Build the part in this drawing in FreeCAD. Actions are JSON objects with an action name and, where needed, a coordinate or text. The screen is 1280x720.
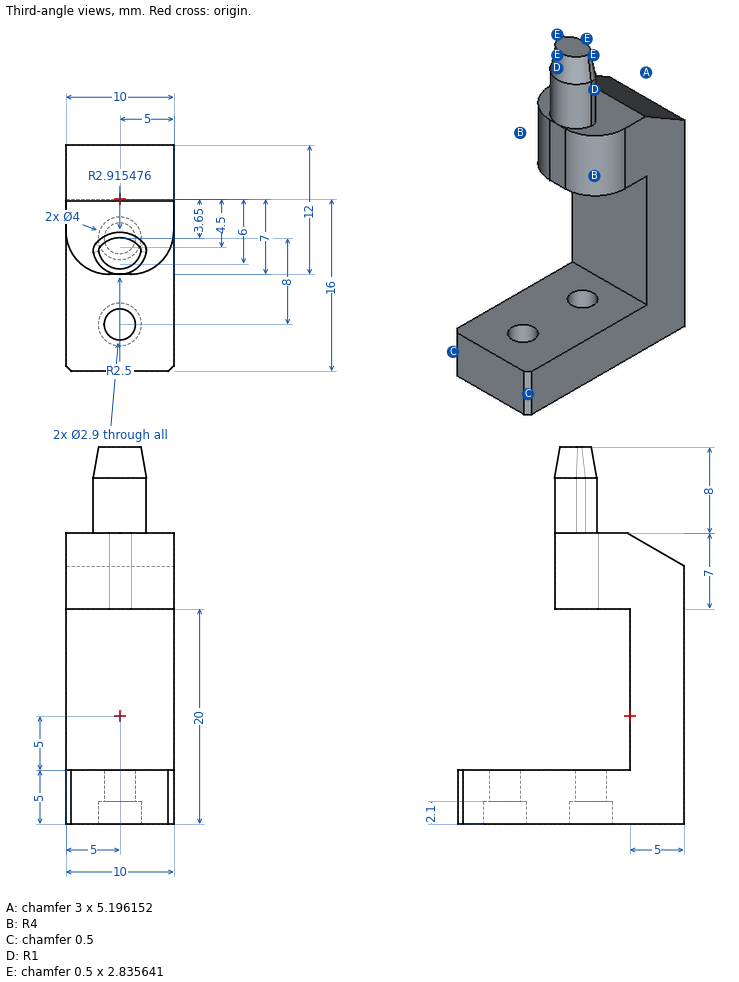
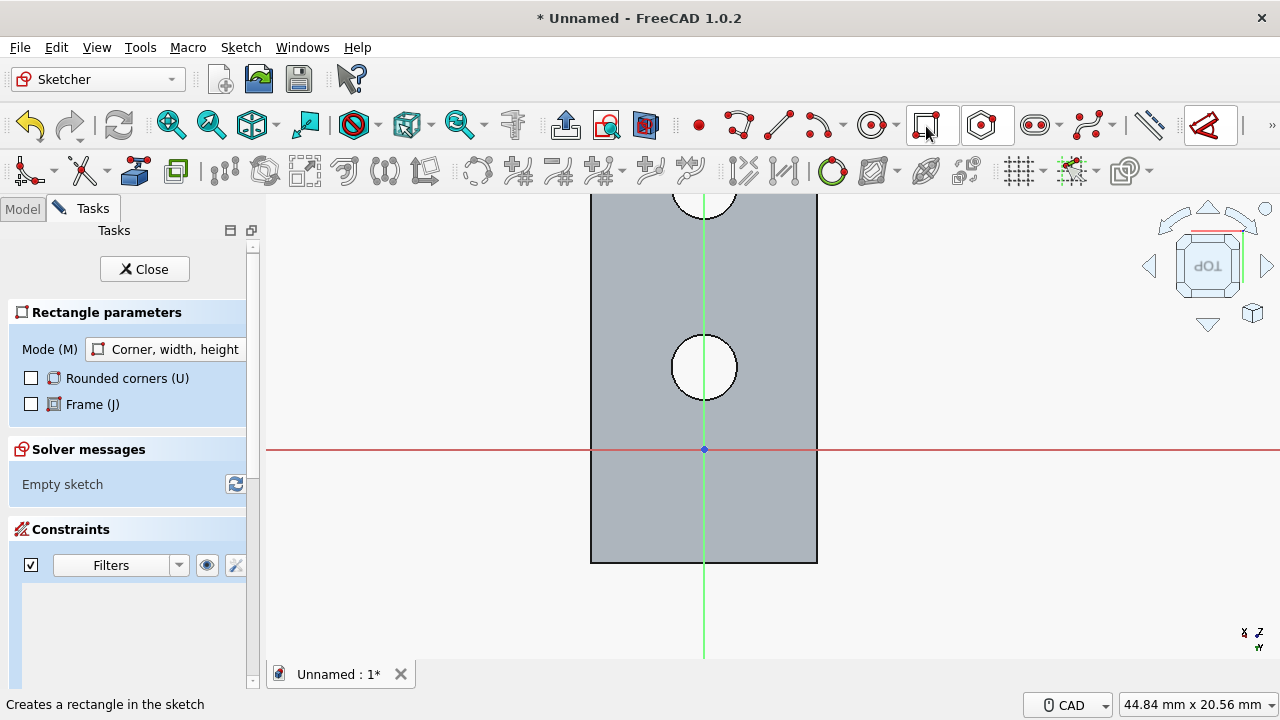
{"action": "left_click", "coordinate": [591, 292]}
{"action": "left_click", "coordinate": [817, 563]}
{"action": "key", "text": "Escape"}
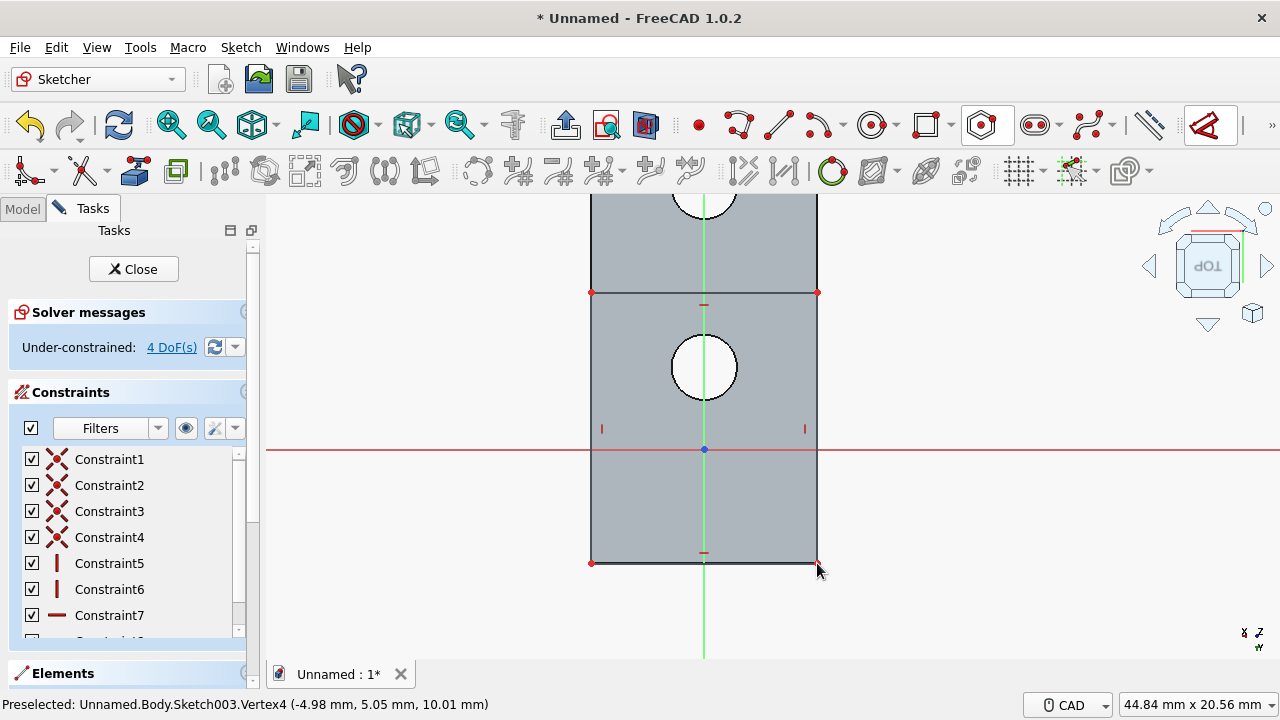
{"action": "left_click", "coordinate": [1204, 126]}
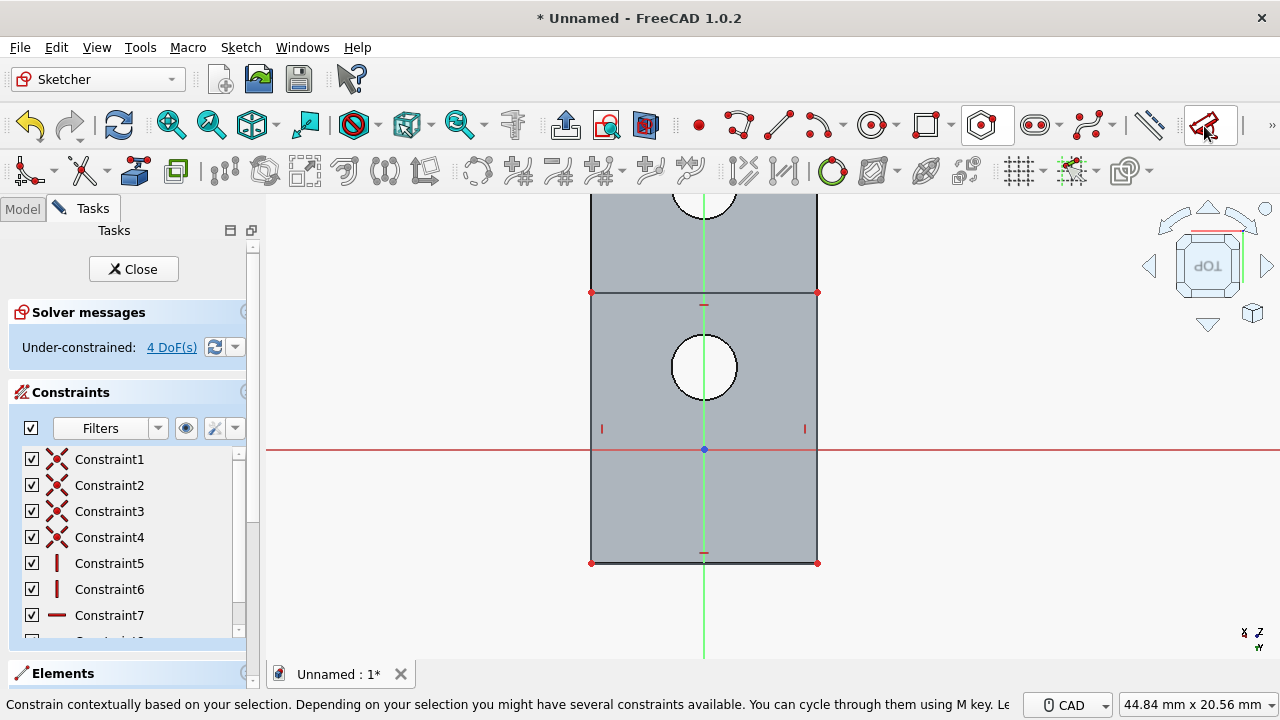
{"action": "left_click", "coordinate": [591, 374]}
{"action": "left_click", "coordinate": [557, 428]}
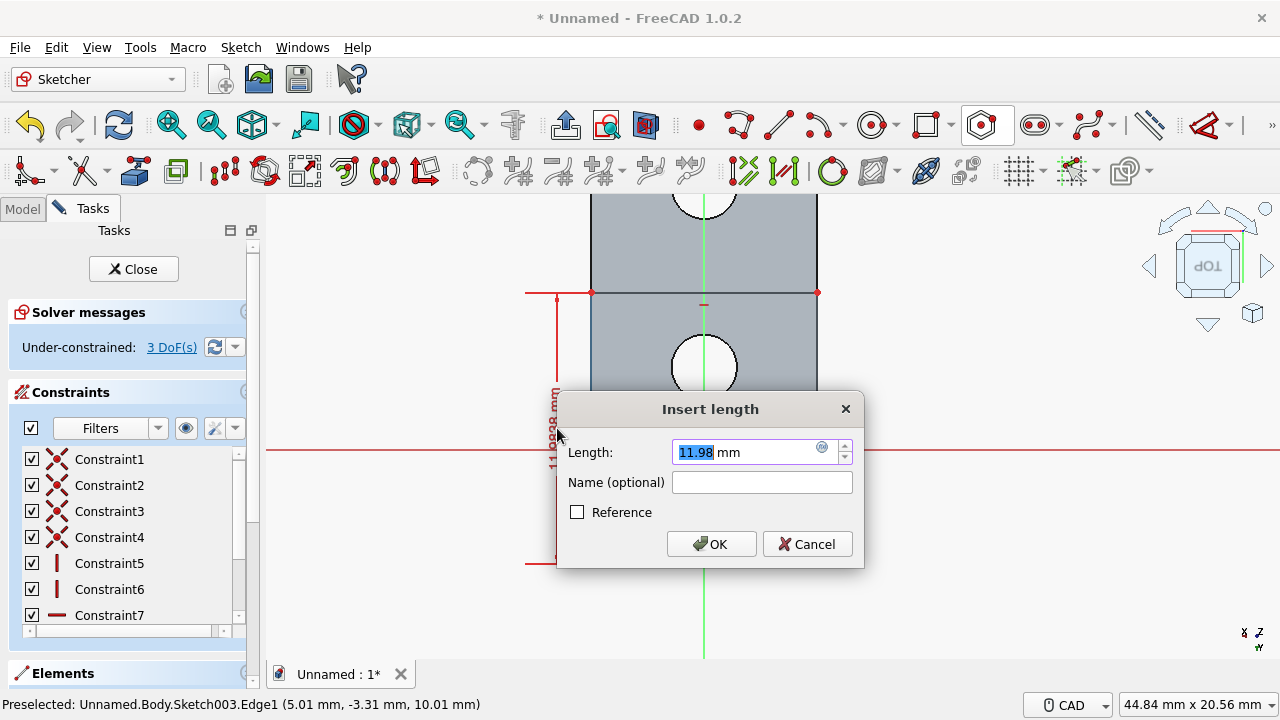
{"action": "type", "text": "12"}
{"action": "key", "text": "Return"}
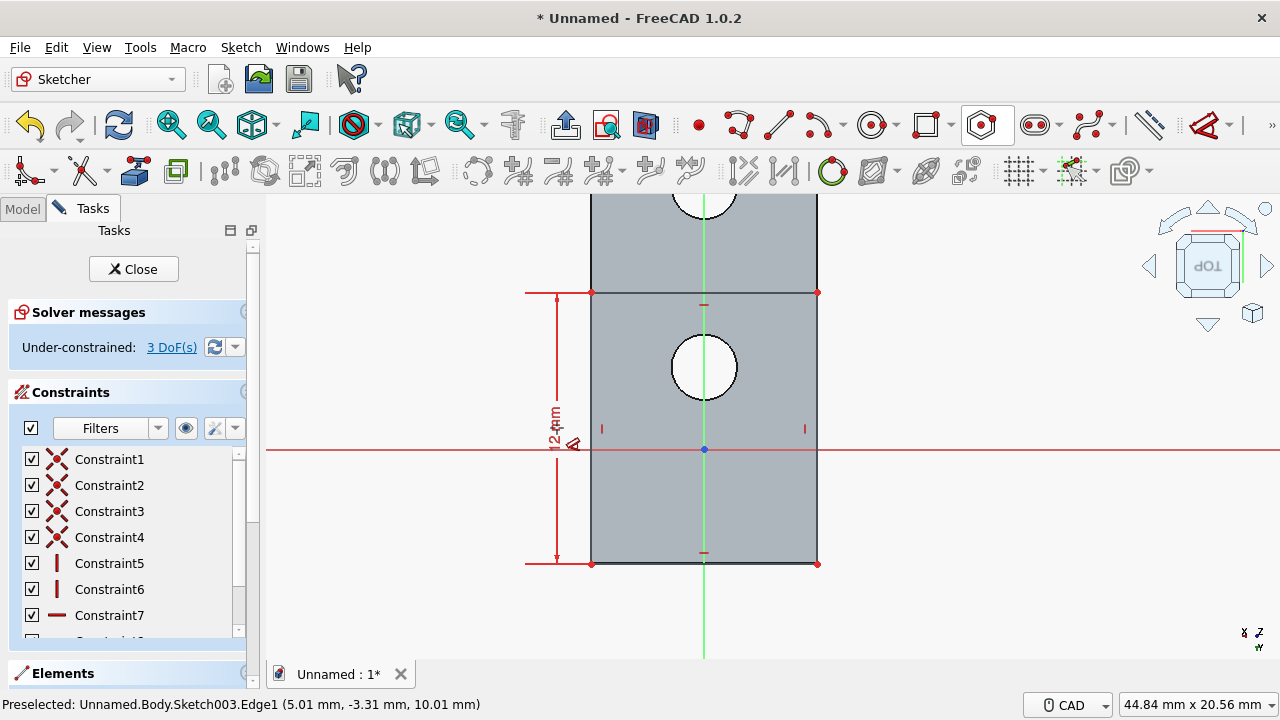
{"action": "left_click", "coordinate": [659, 564]}
{"action": "left_click", "coordinate": [652, 598]}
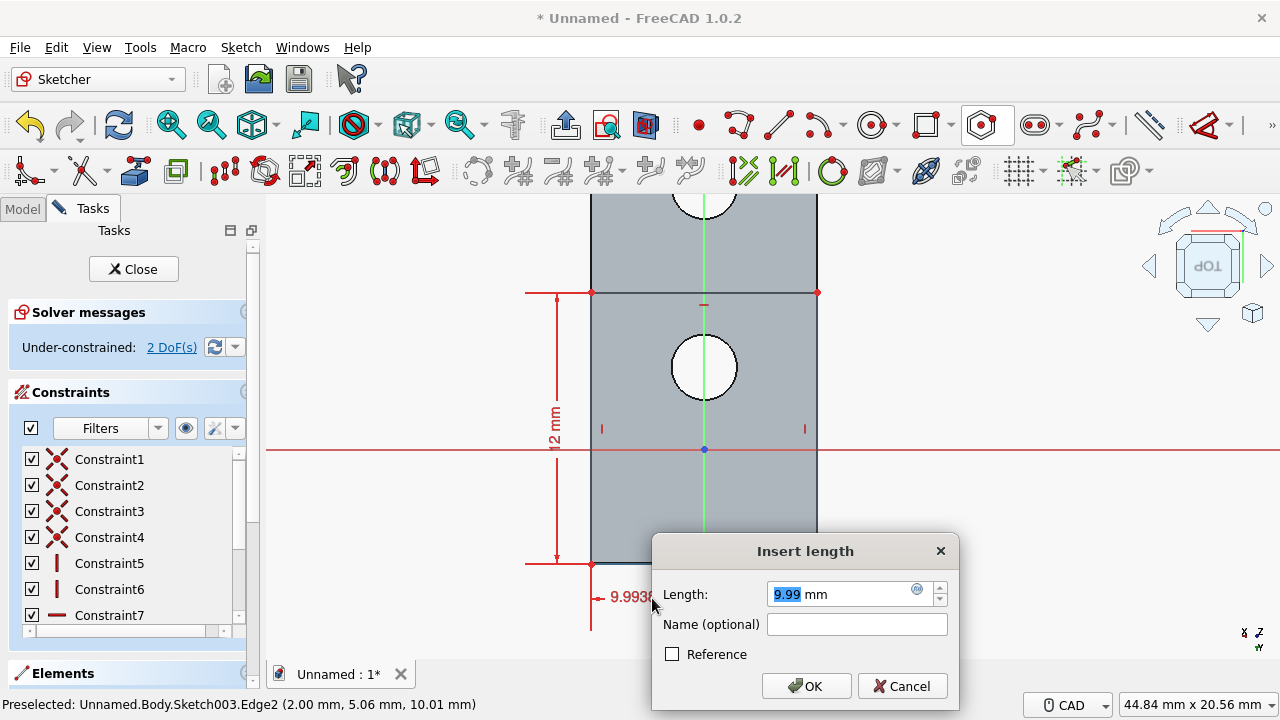
{"action": "type", "text": "10"}
{"action": "key", "text": "Return"}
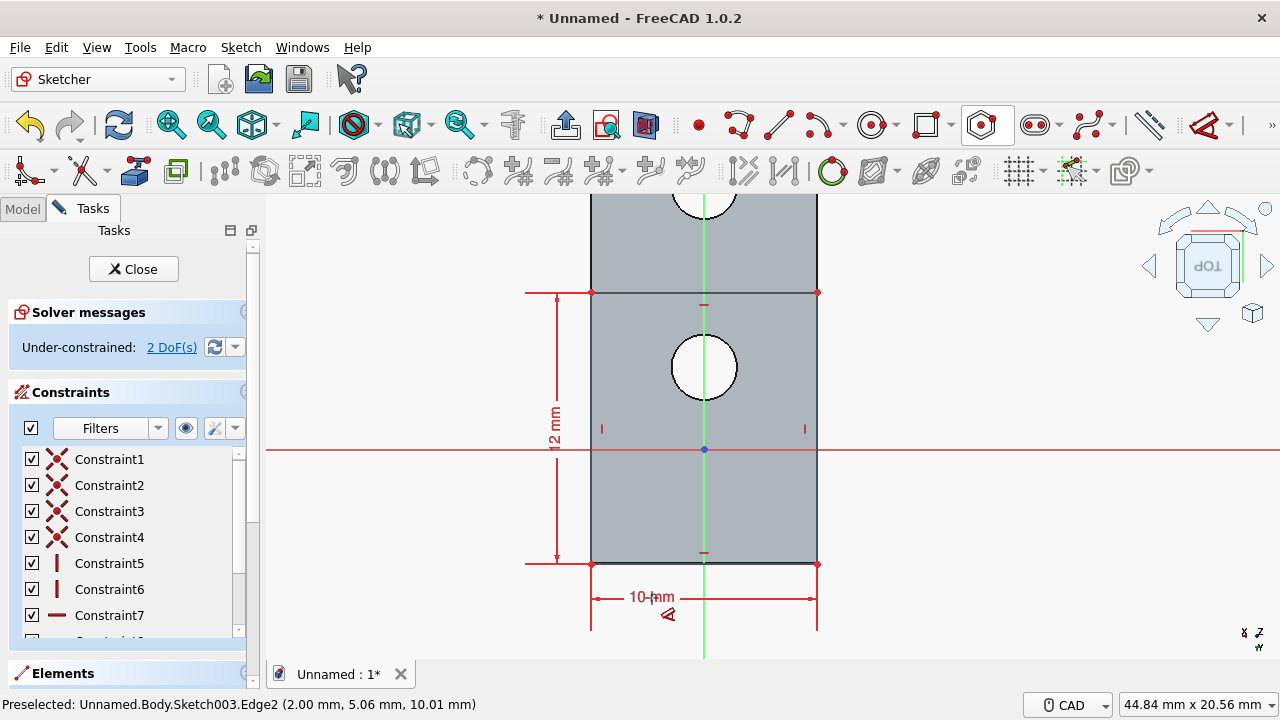
{"action": "left_click", "coordinate": [591, 293]}
{"action": "left_click", "coordinate": [648, 259]}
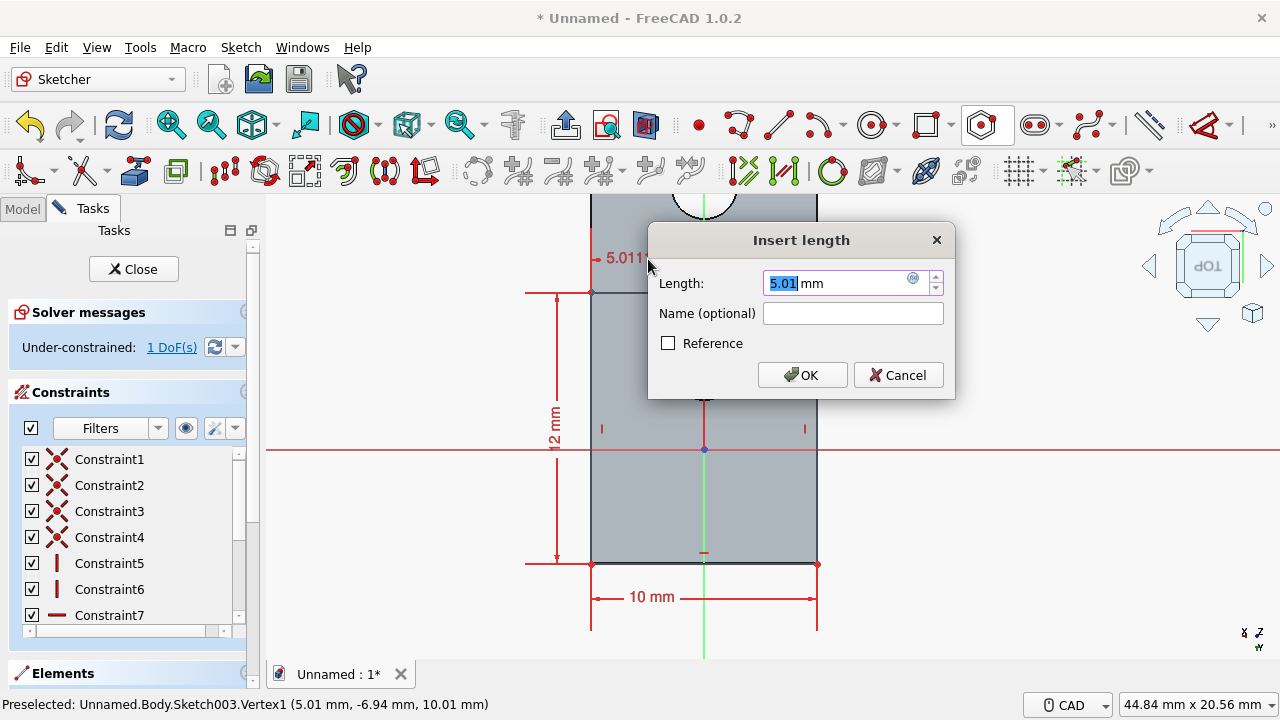
{"action": "type", "text": "5"}
{"action": "key", "text": "Return"}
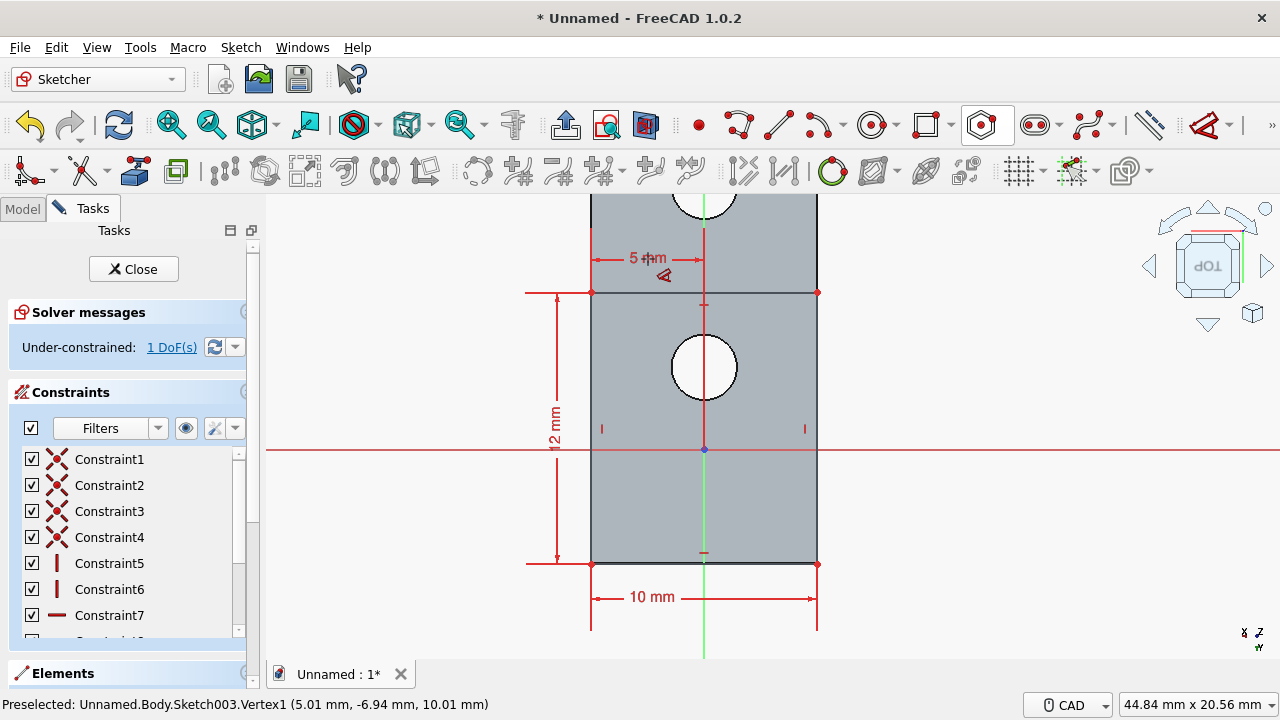
{"action": "left_click", "coordinate": [591, 293]}
{"action": "left_click", "coordinate": [557, 371]}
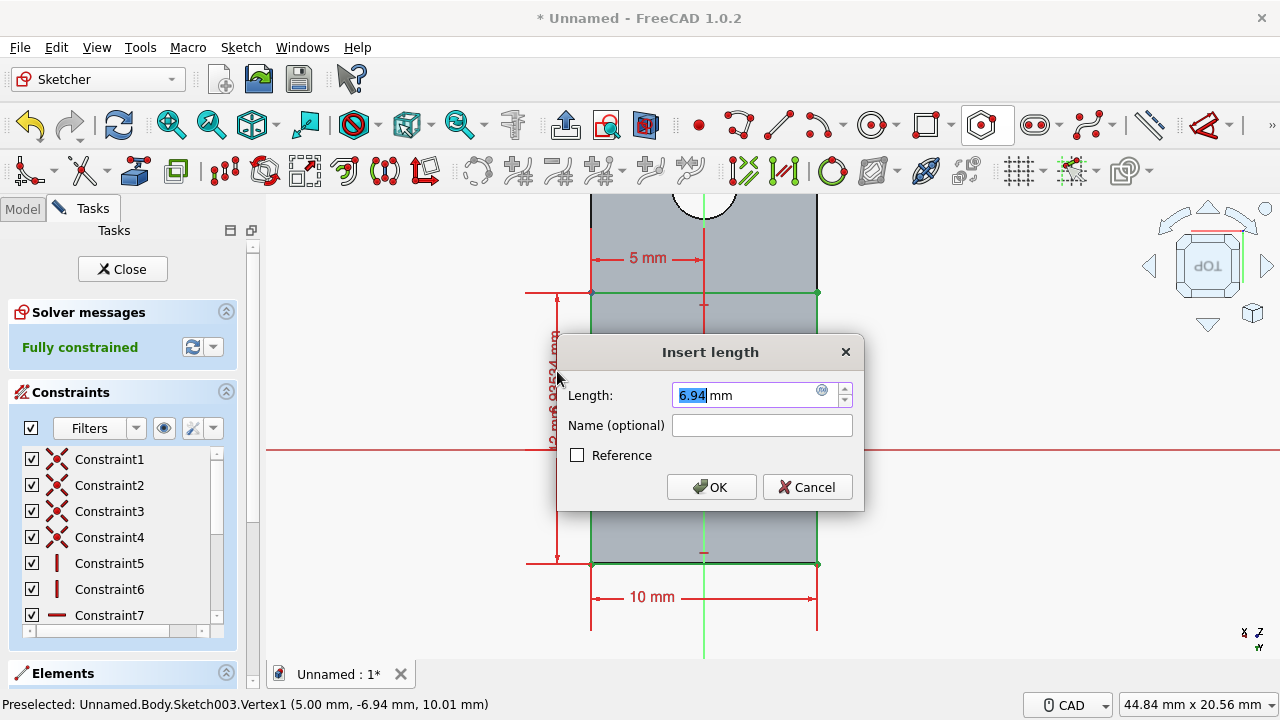
{"action": "type", "text": "7"}
{"action": "key", "text": "Return"}
{"action": "key", "text": "Escape"}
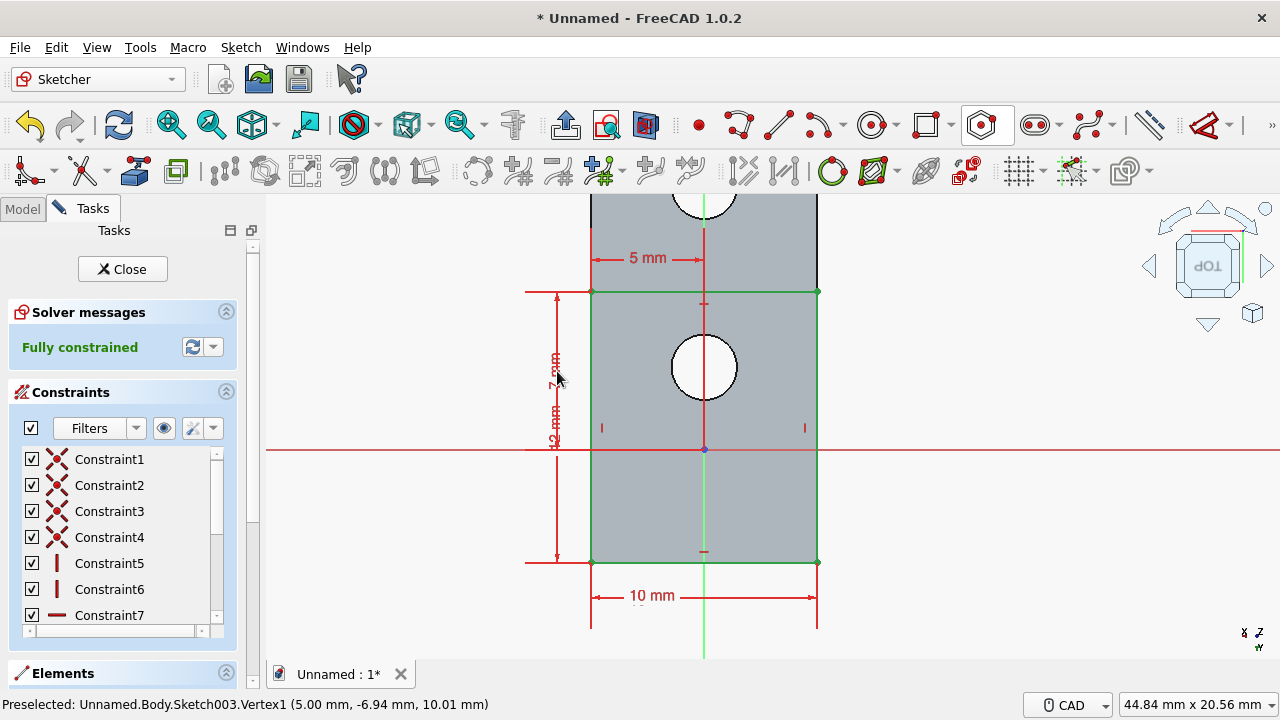
{"action": "left_click", "coordinate": [123, 269]}